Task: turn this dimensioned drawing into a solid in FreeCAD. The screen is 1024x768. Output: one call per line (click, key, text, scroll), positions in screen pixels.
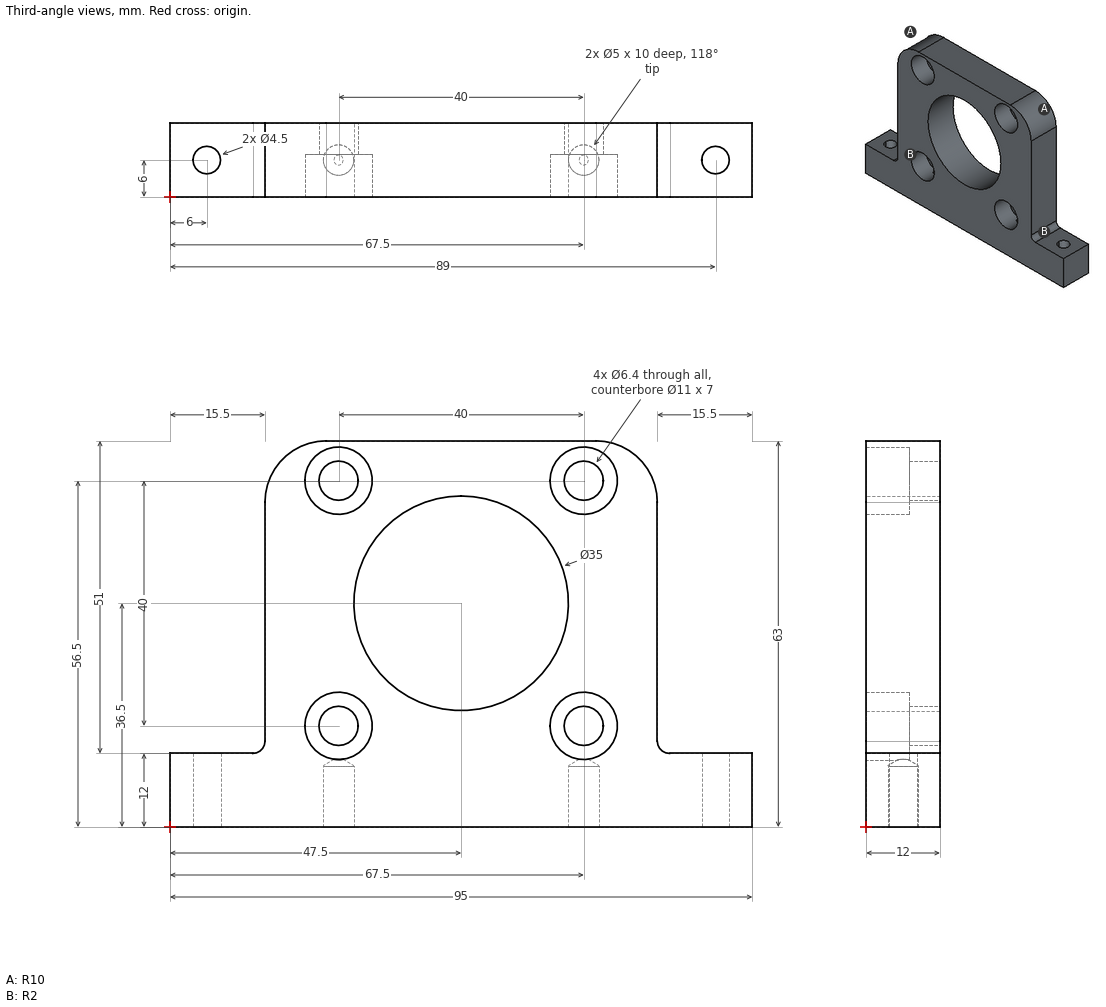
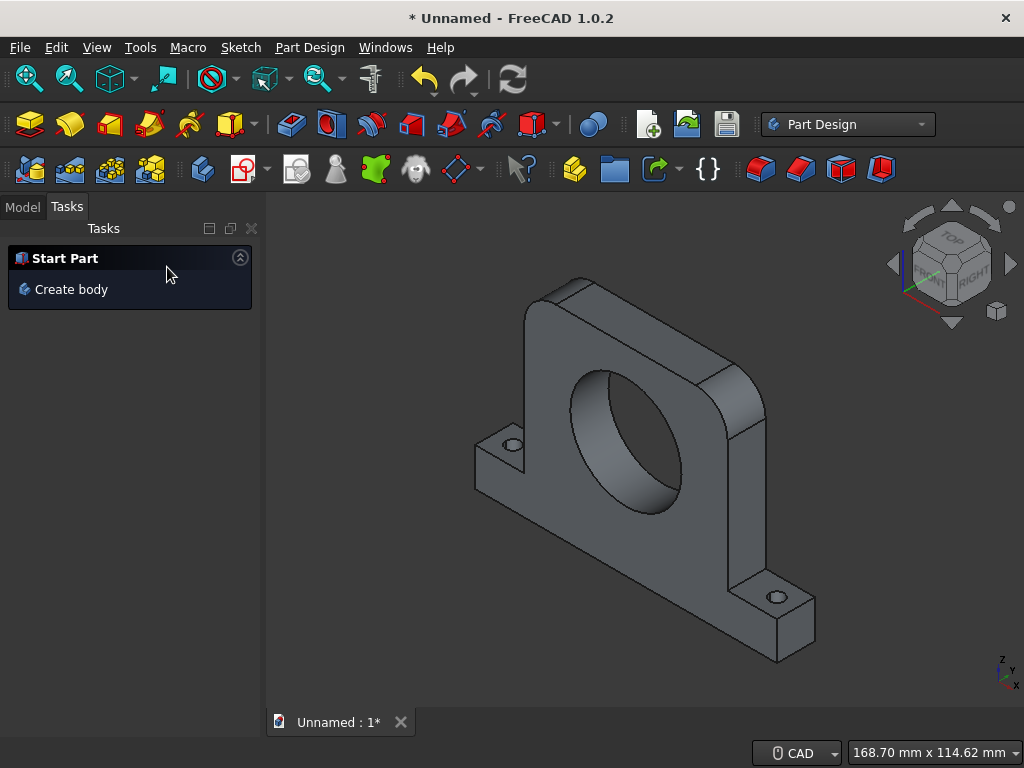
key(2)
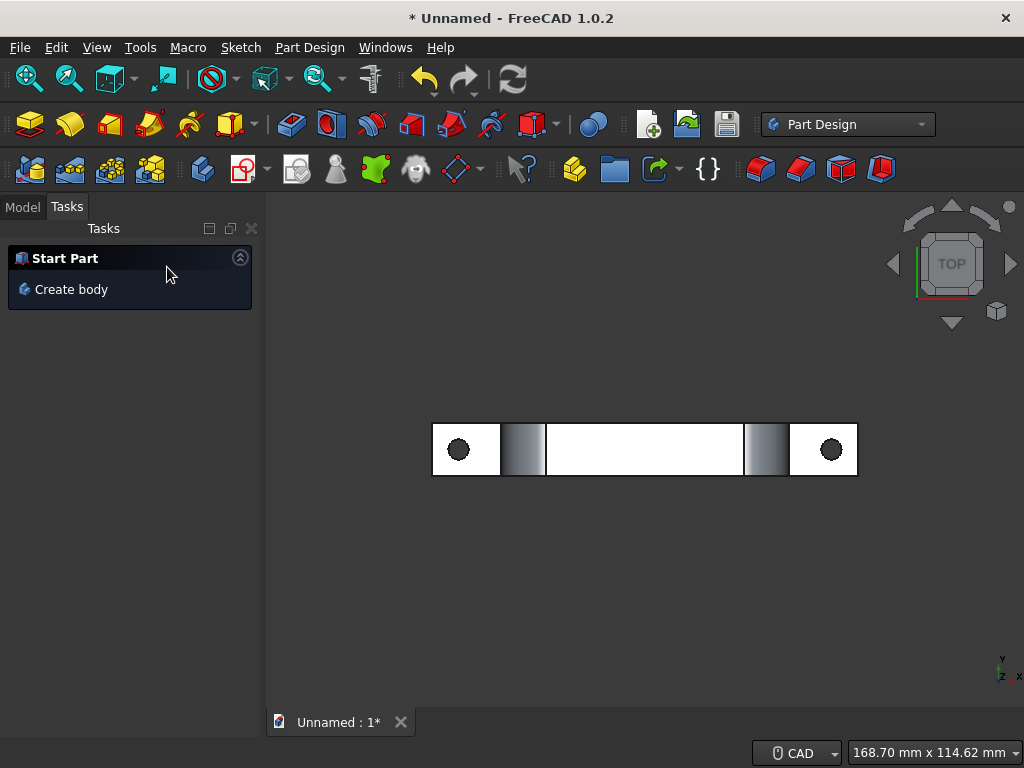
key(1)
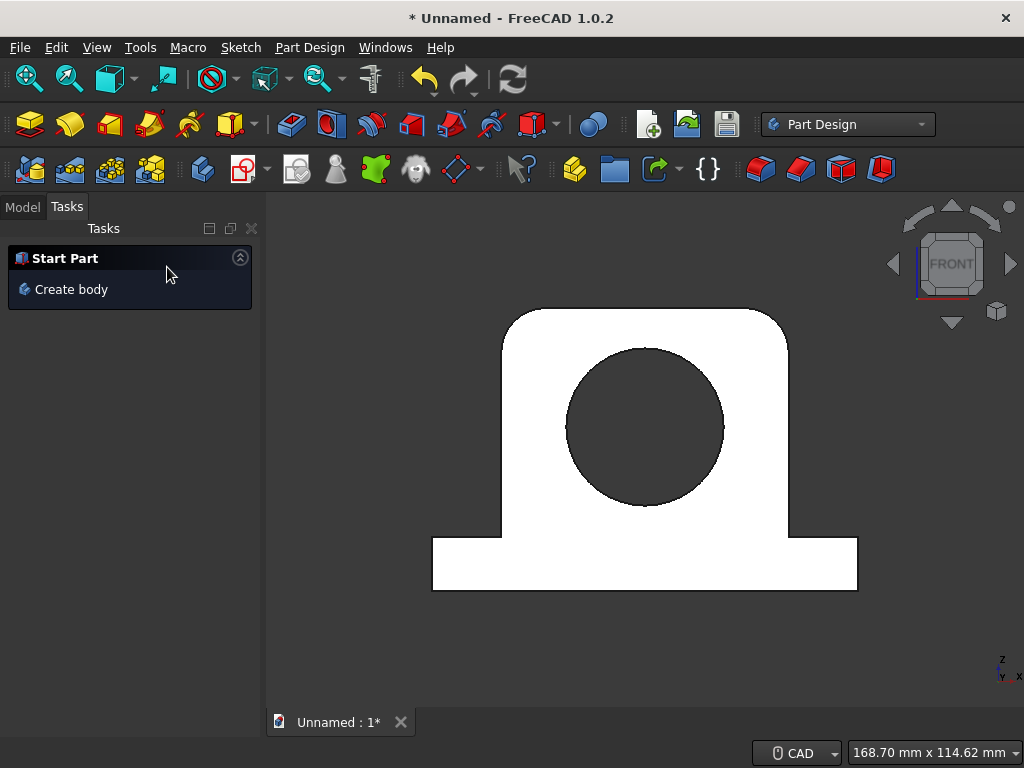
key(3)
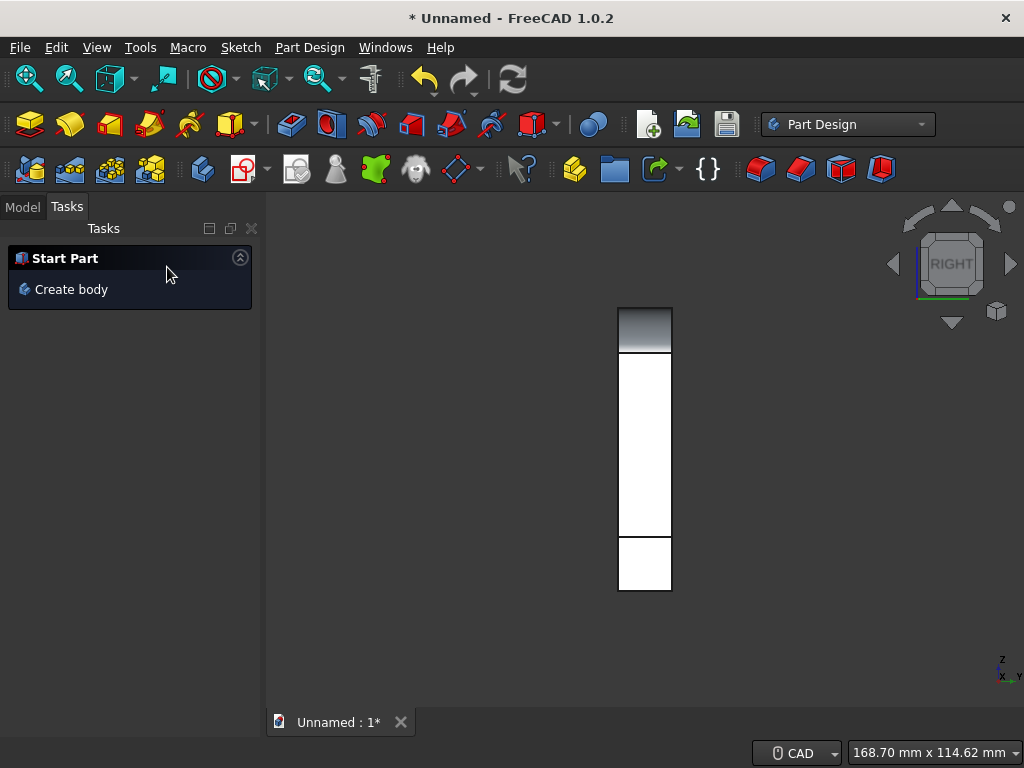
key(5)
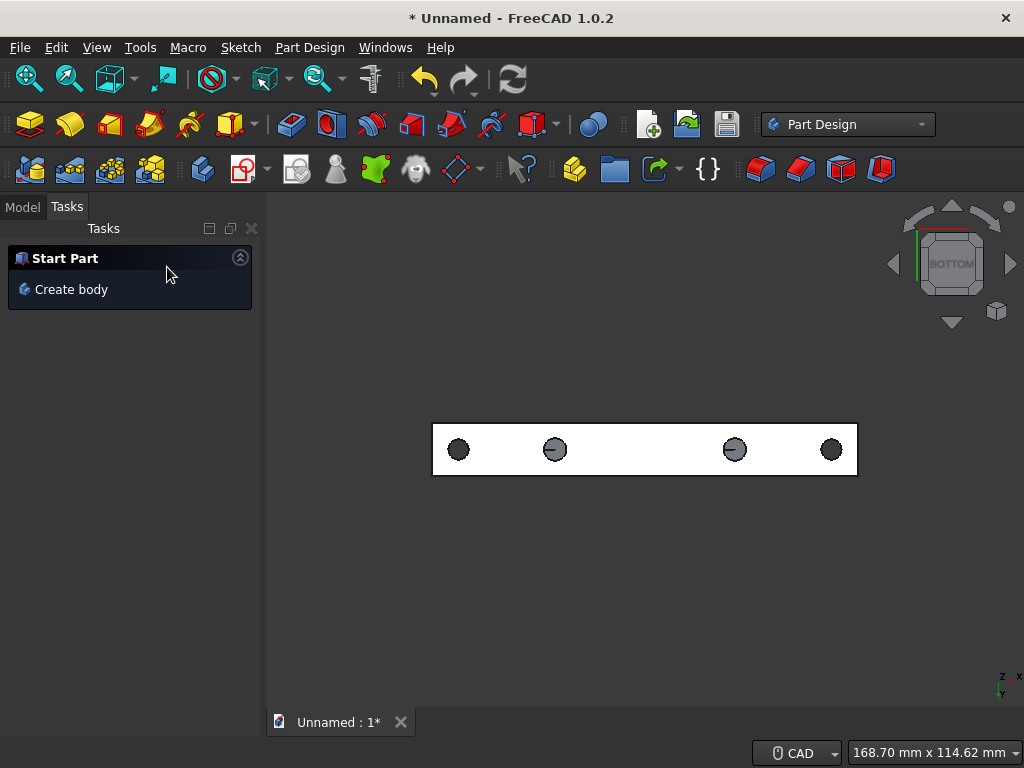
key(4)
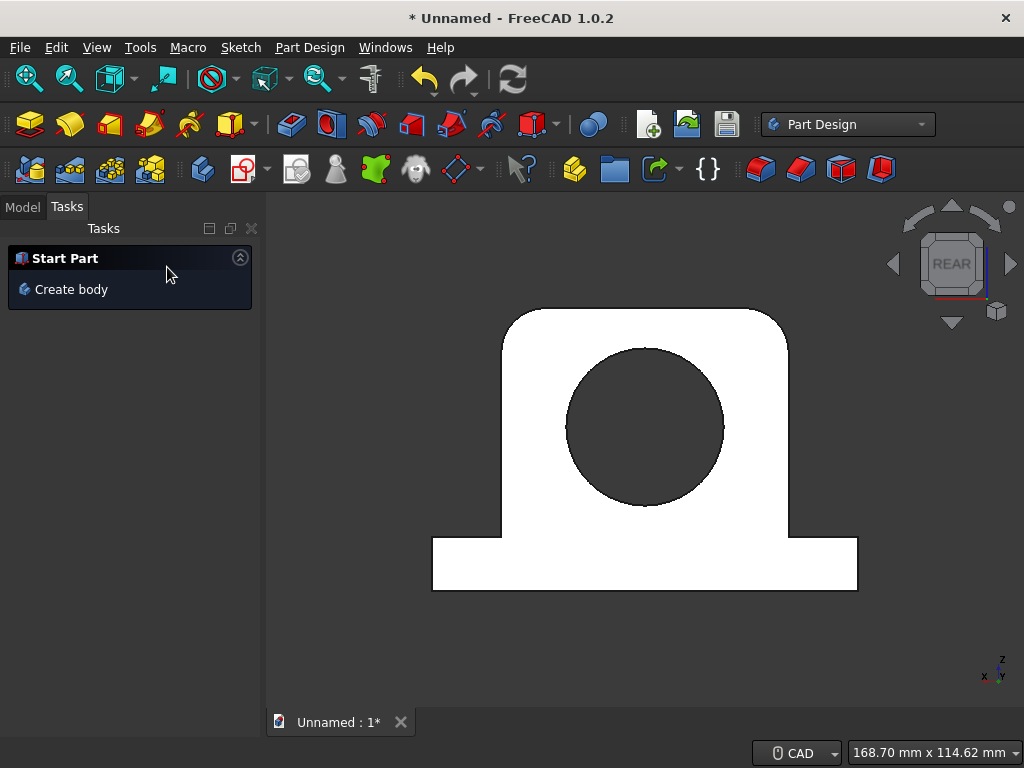
key(6)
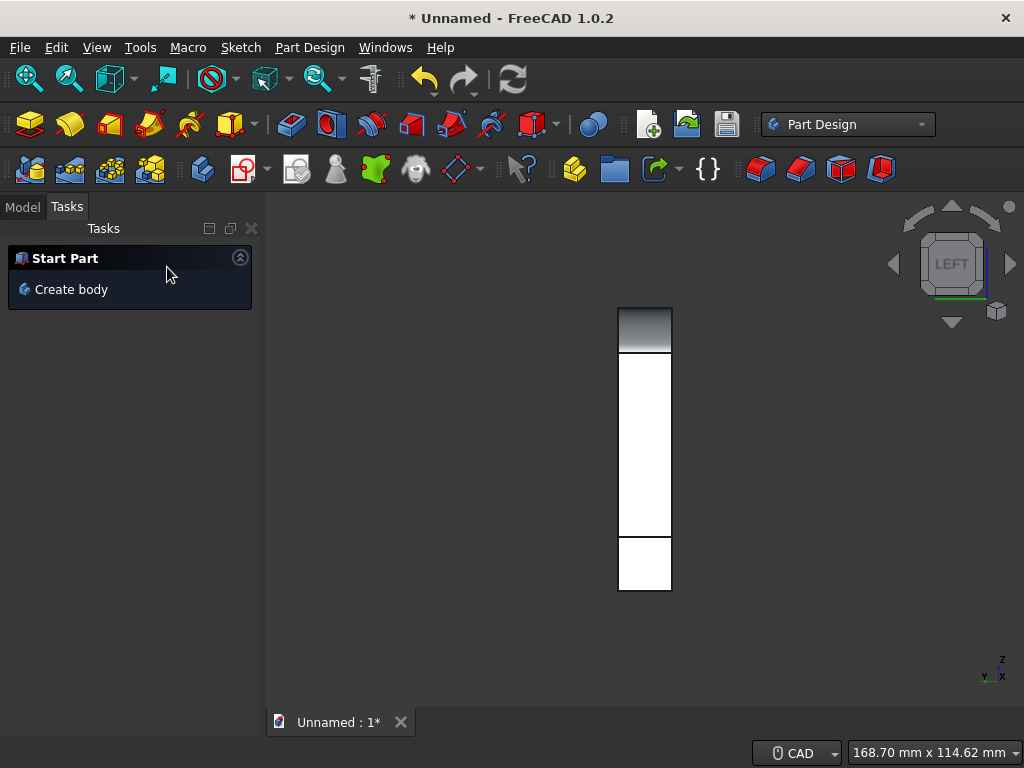
key(v)
key(3)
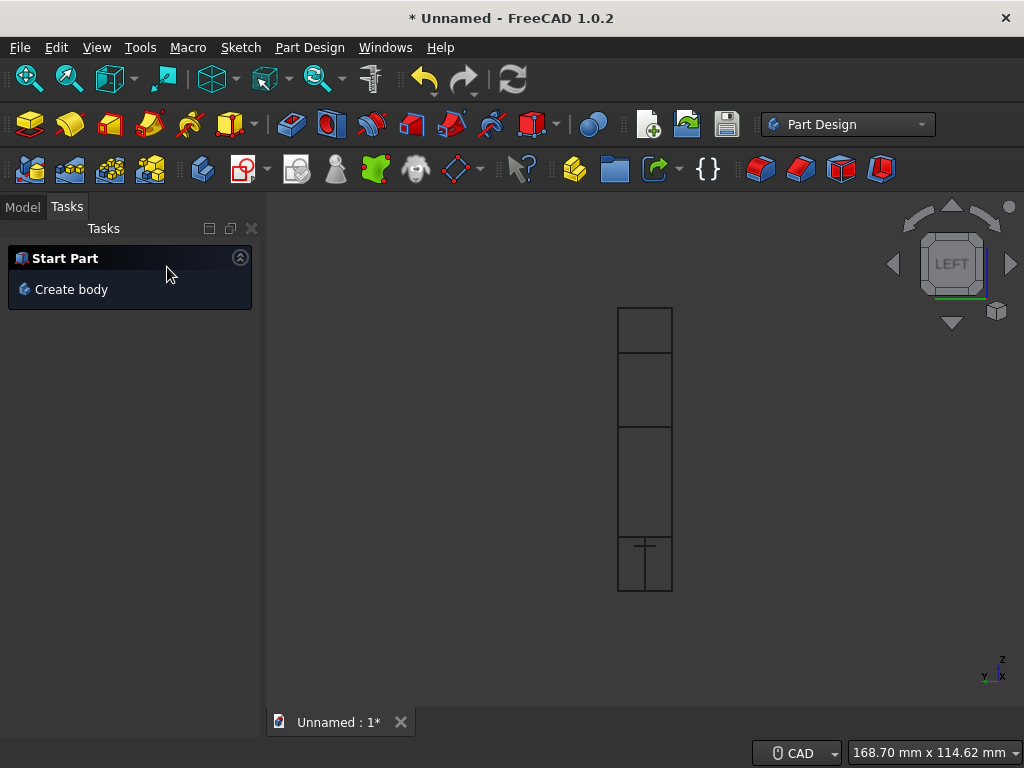
key(0)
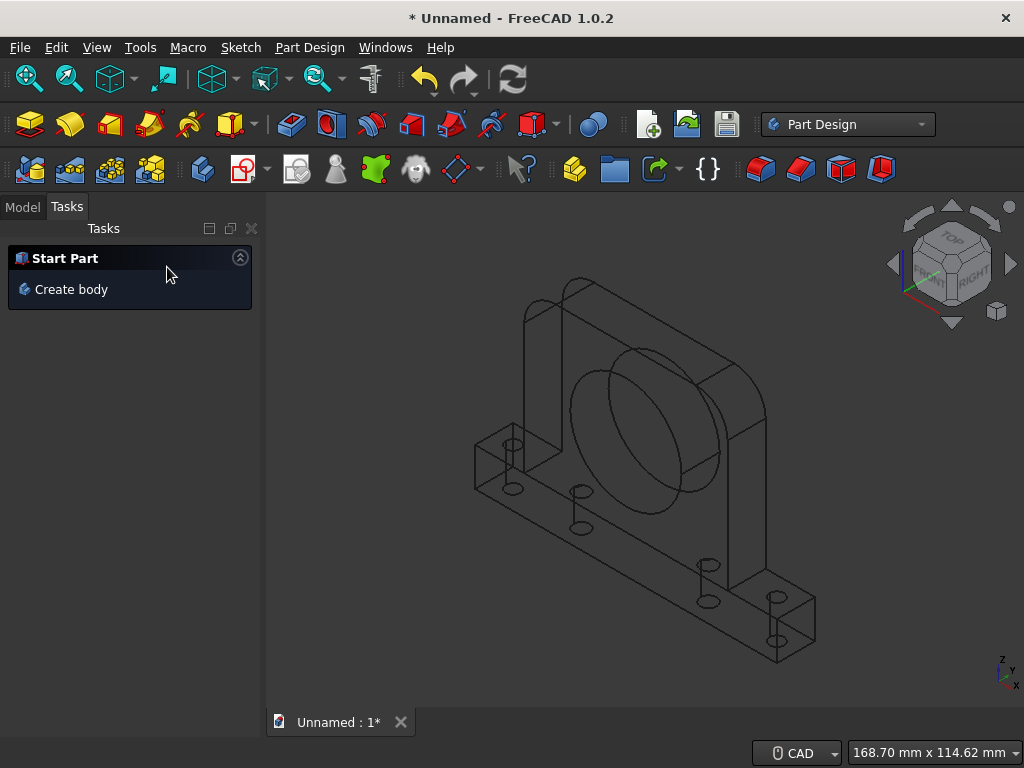
click(543, 461)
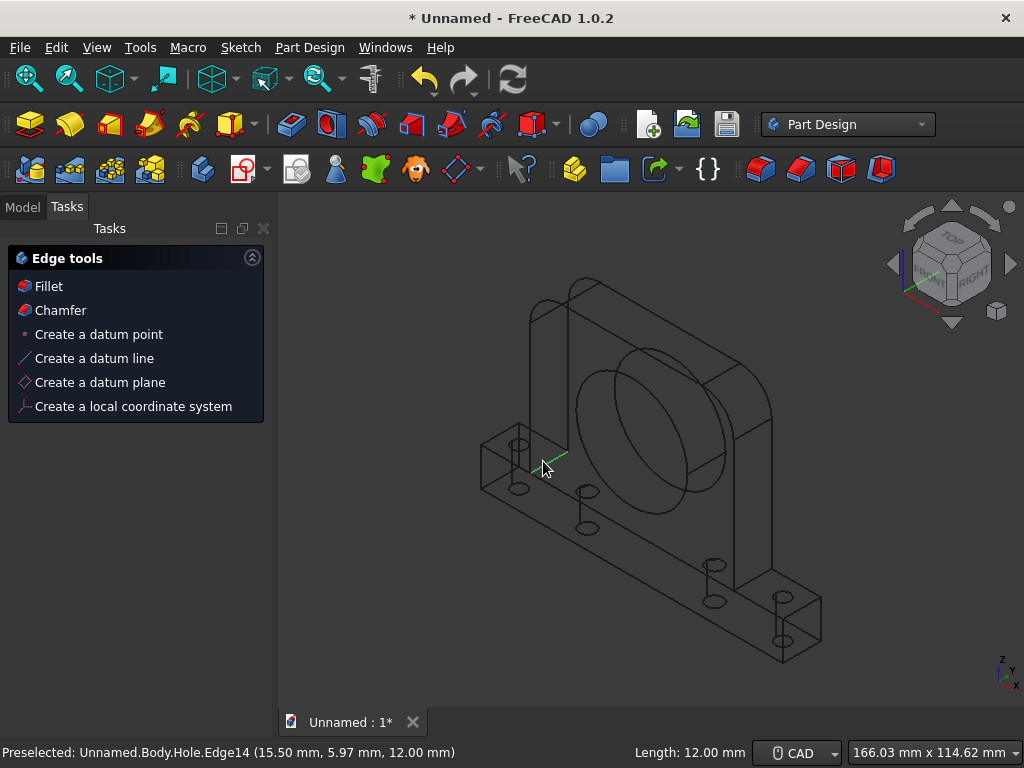
click(753, 579, ctrl)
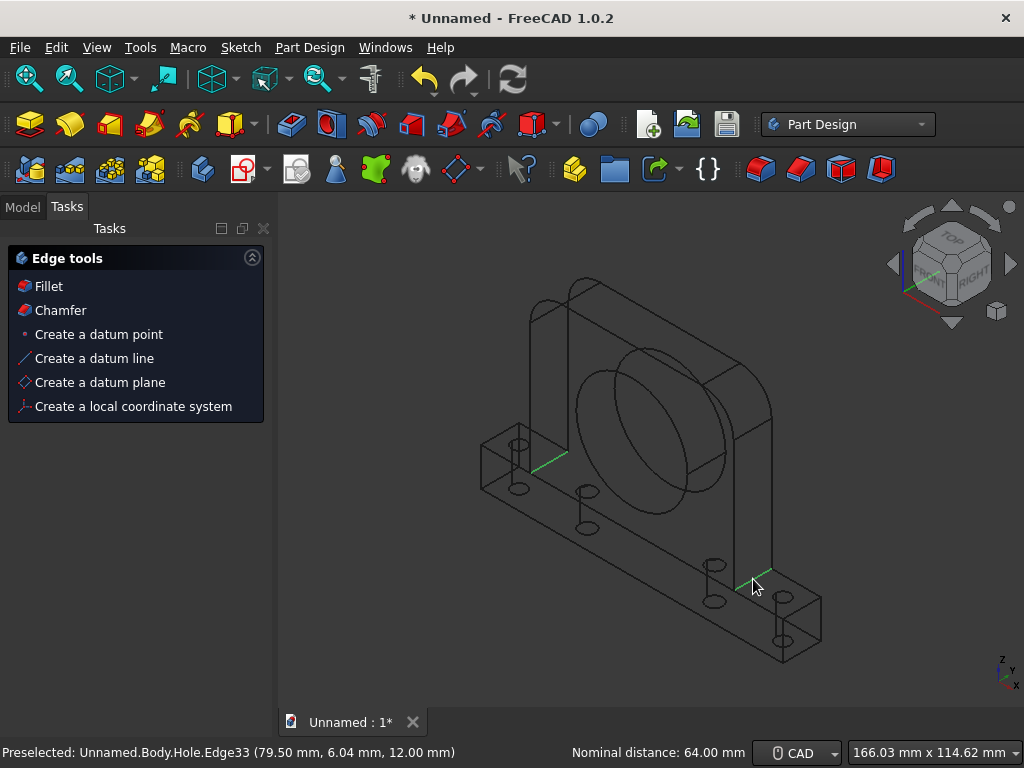
key(v)
key(1)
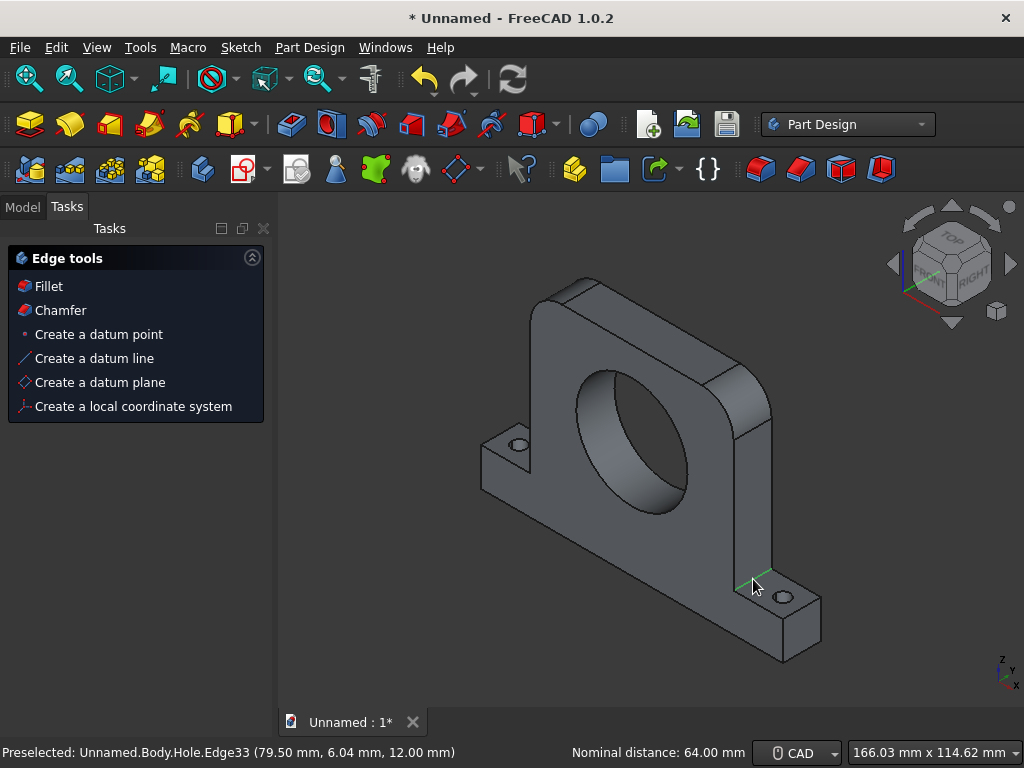
click(762, 170)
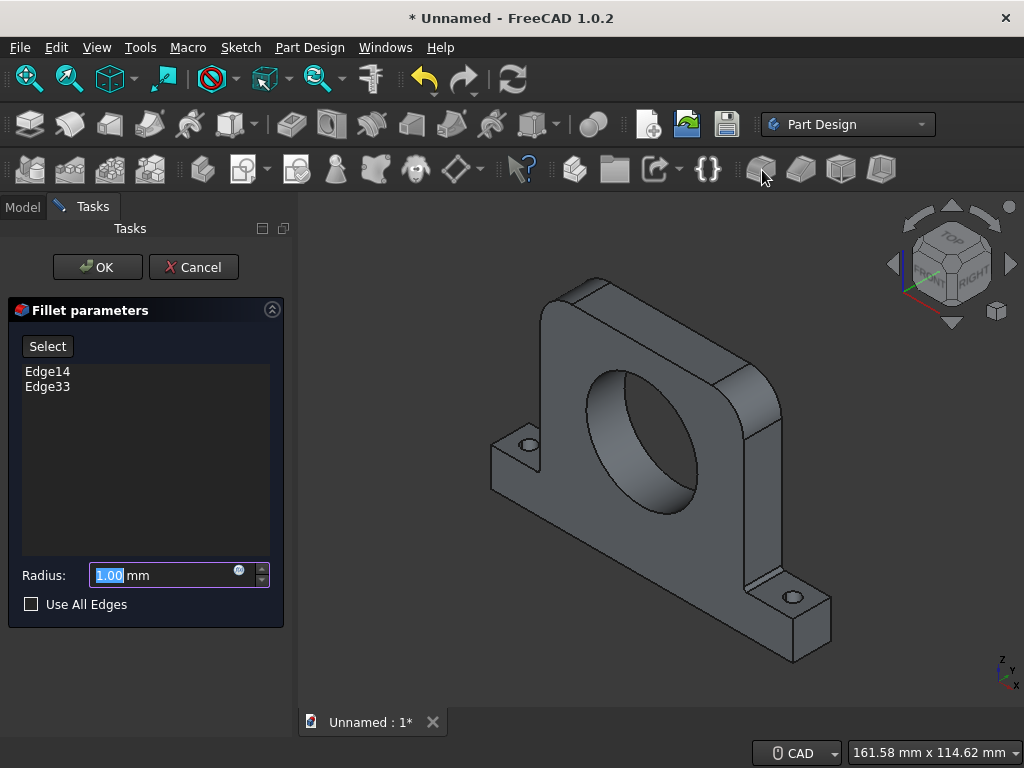
text(2)
key(Tab)